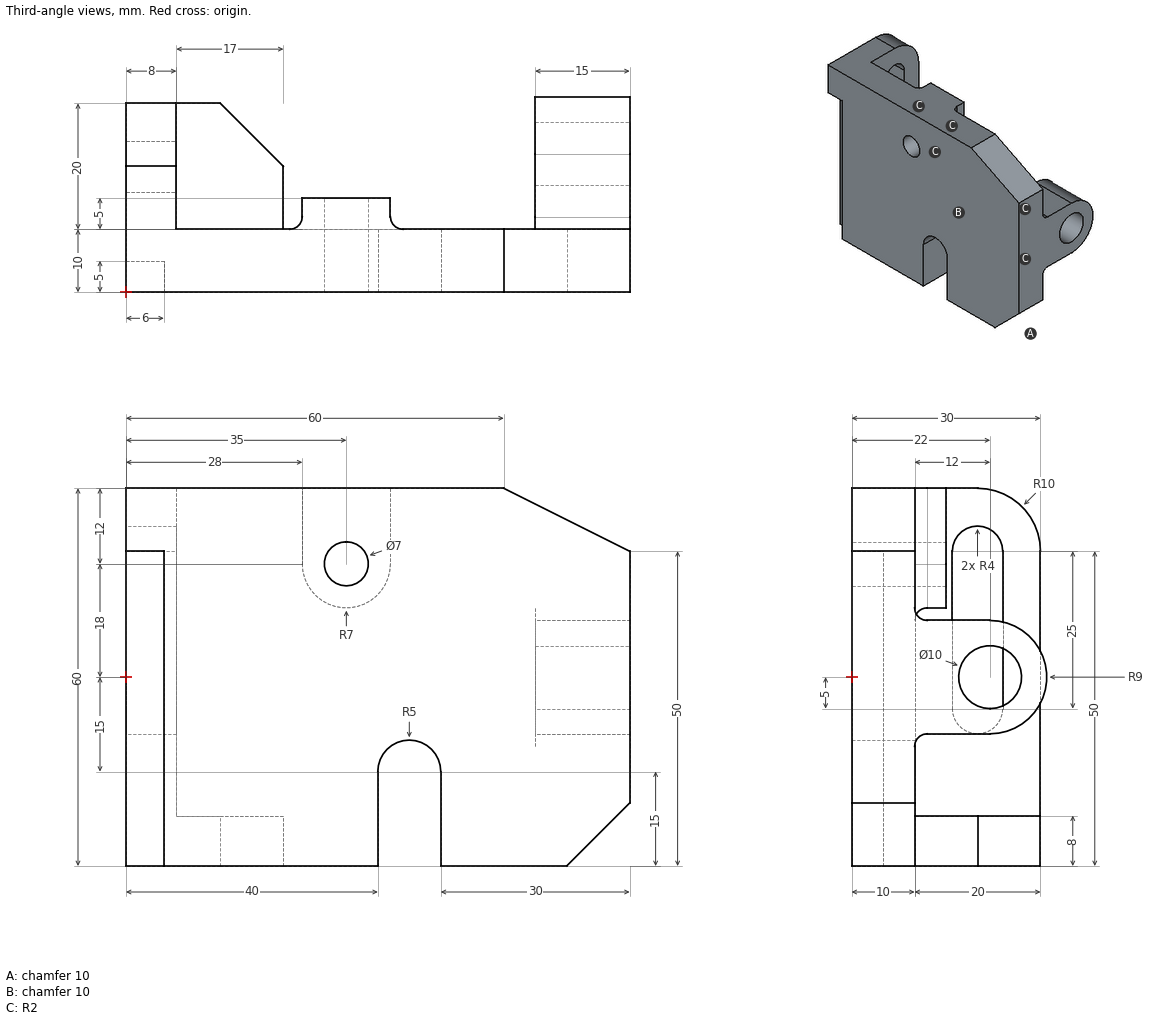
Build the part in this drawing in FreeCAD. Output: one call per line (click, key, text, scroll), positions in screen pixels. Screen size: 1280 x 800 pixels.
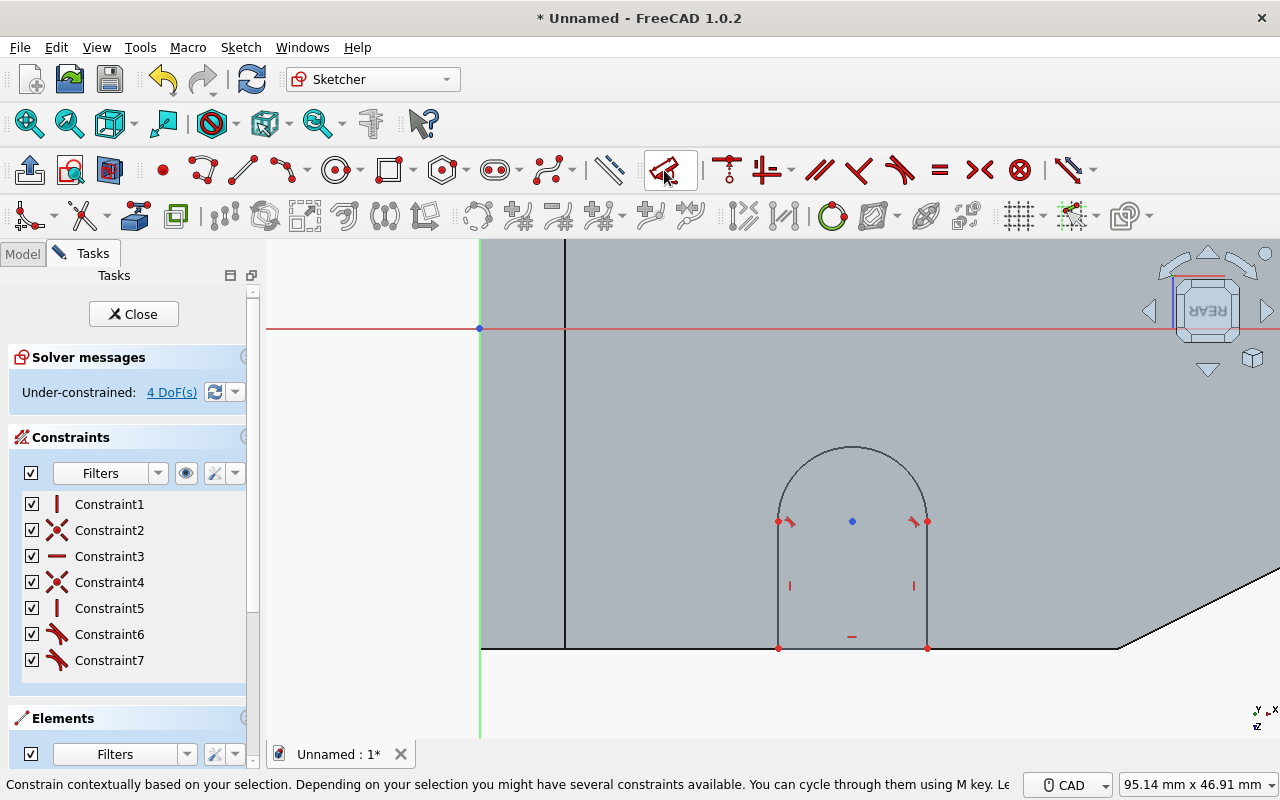
click(896, 461)
click(915, 435)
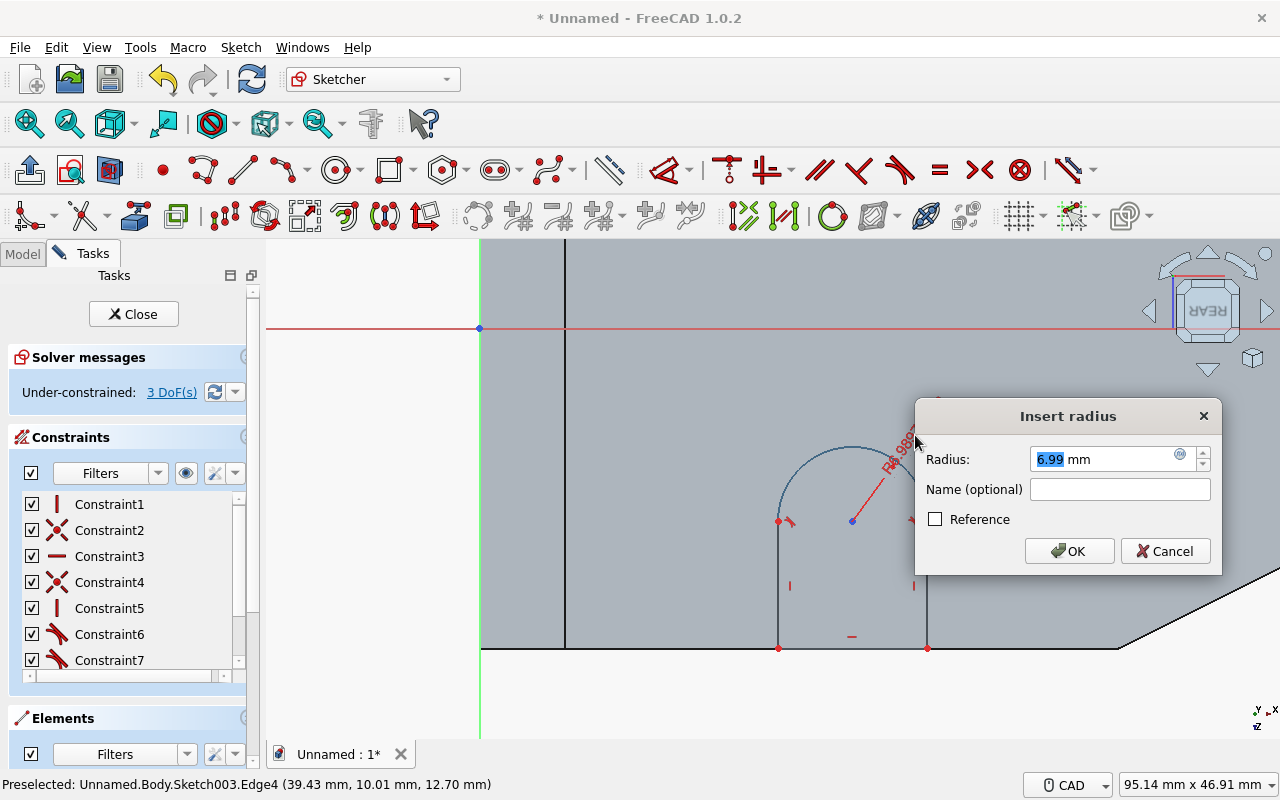
text(7)
key(Return)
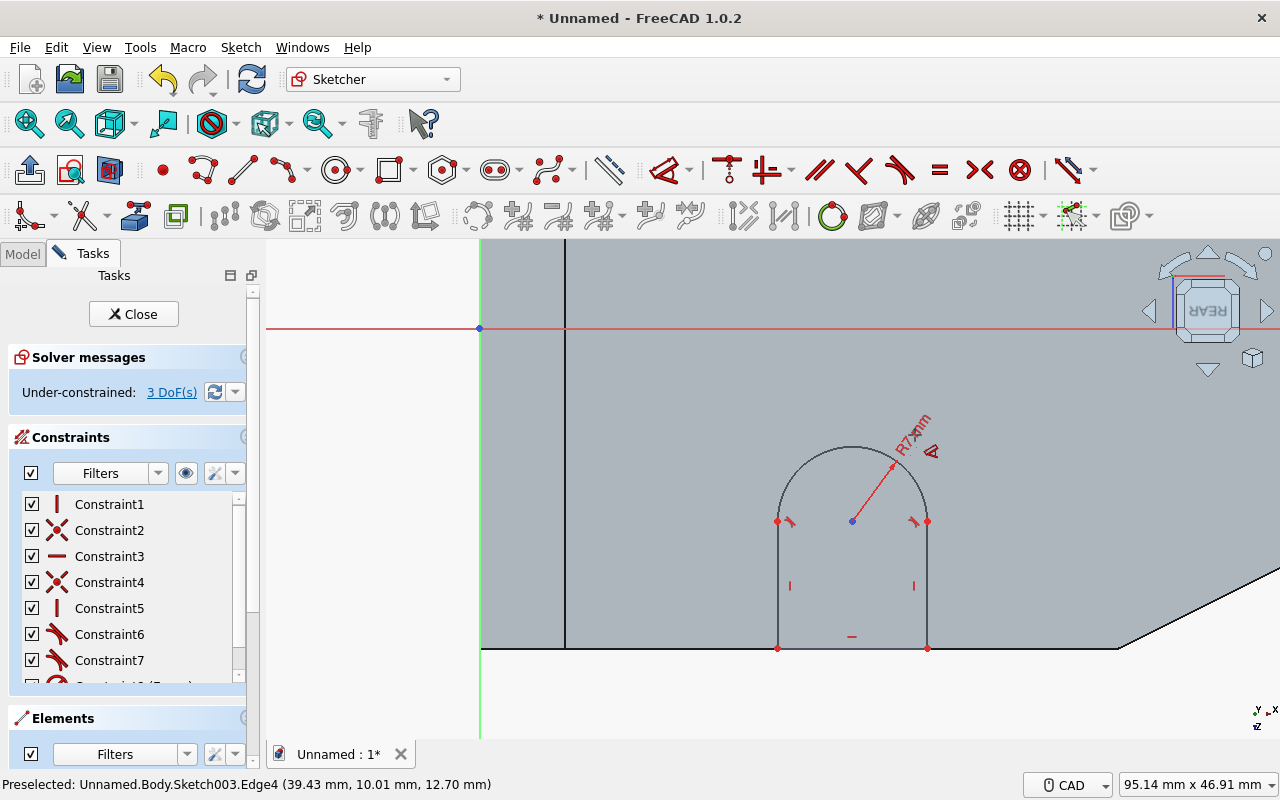
click(778, 560)
click(812, 585)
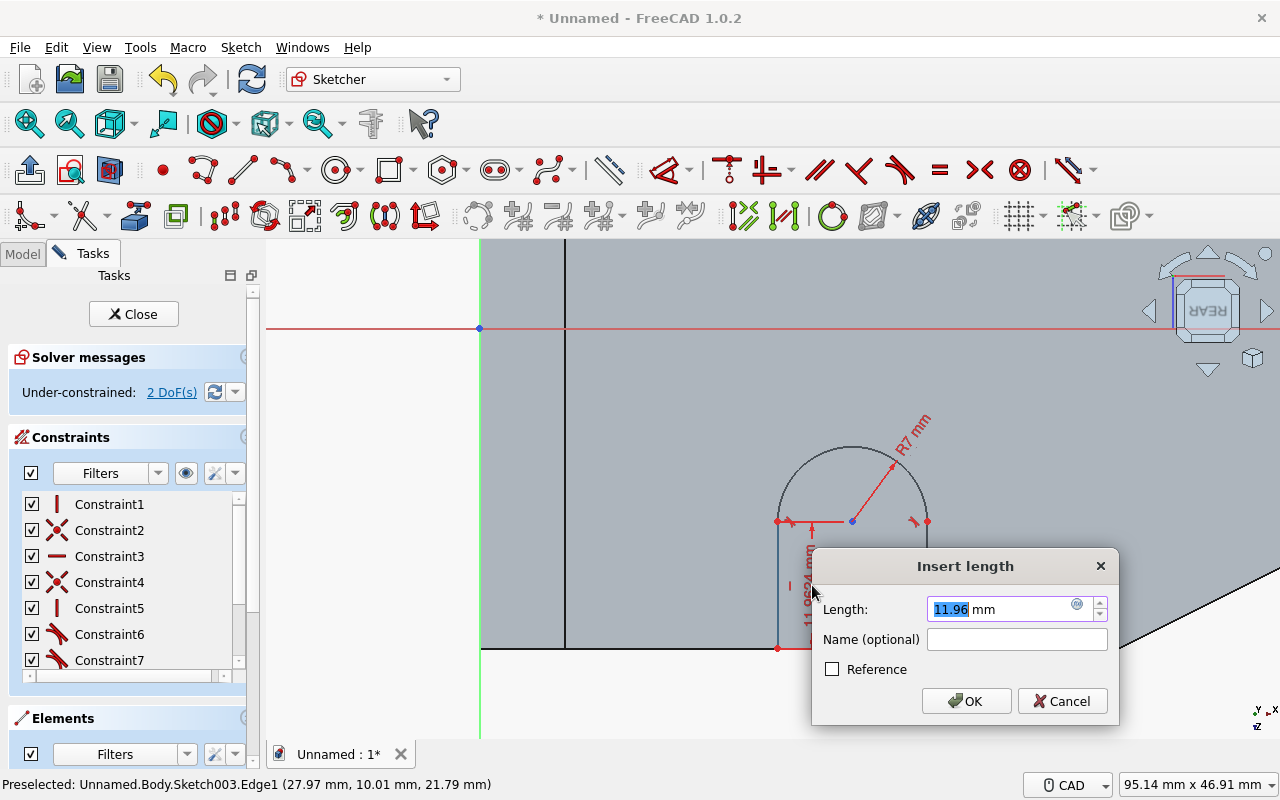
text(12)
key(Return)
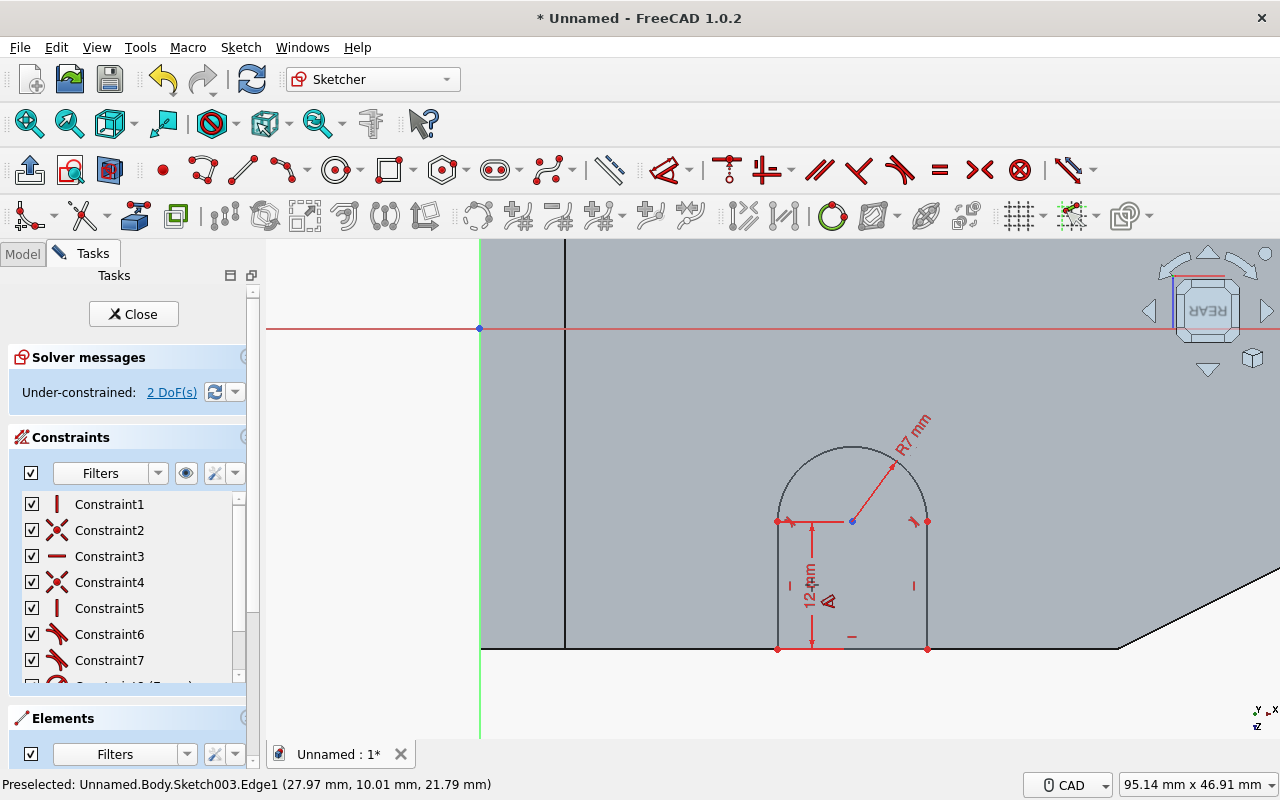
click(778, 522)
click(629, 295)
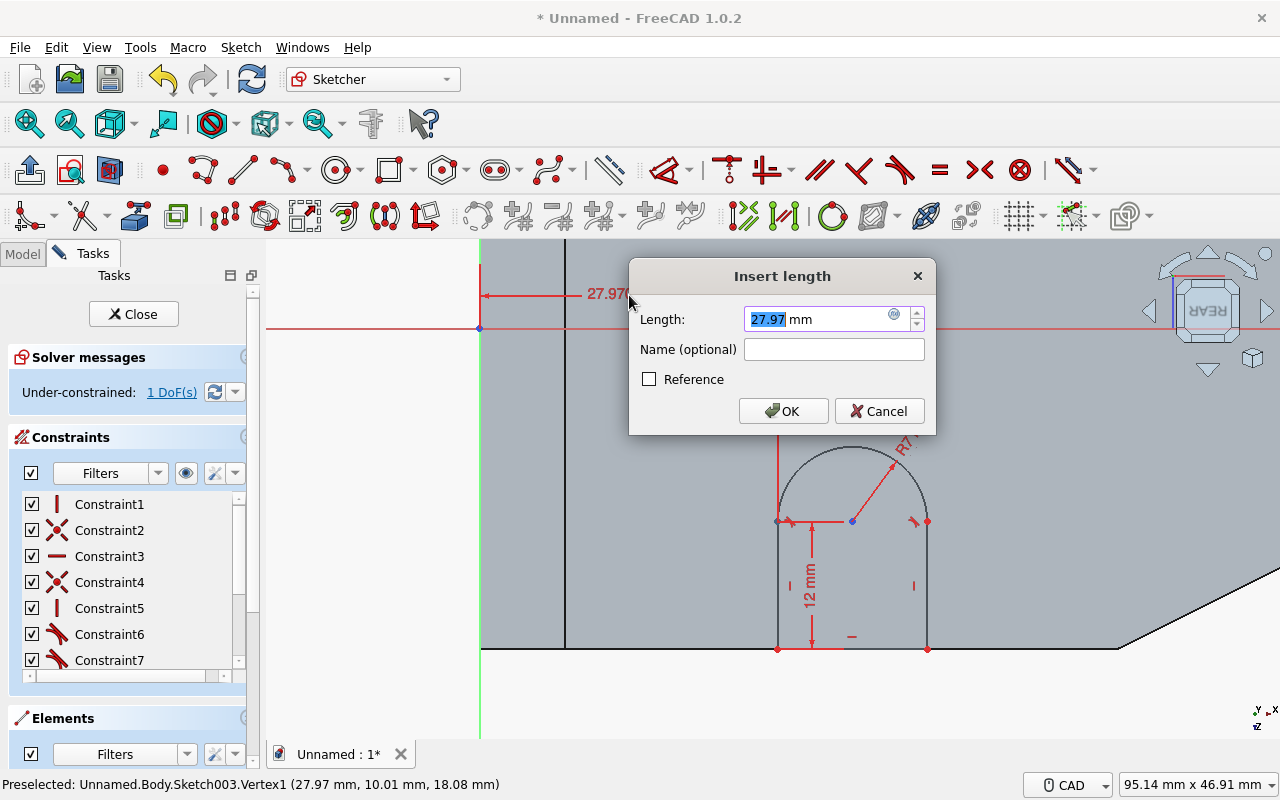
text(28)
key(Return)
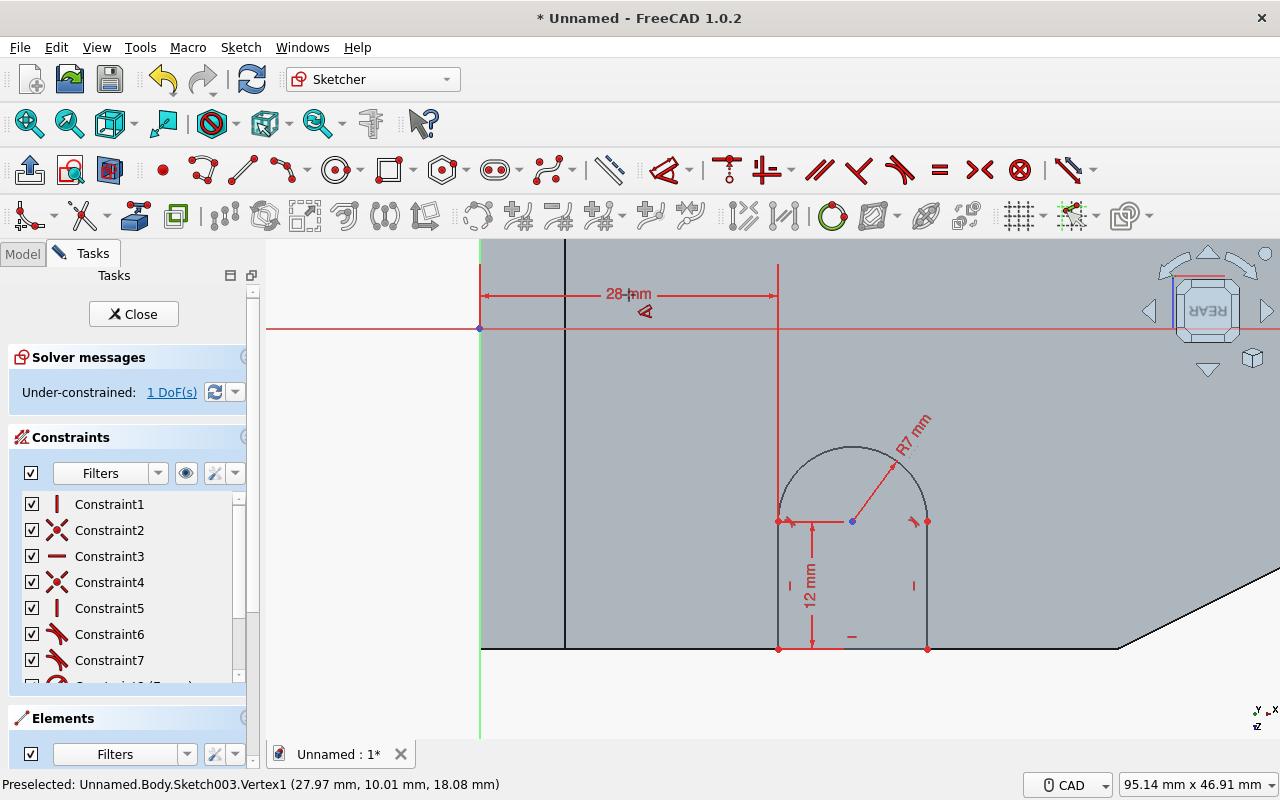
click(778, 522)
click(446, 425)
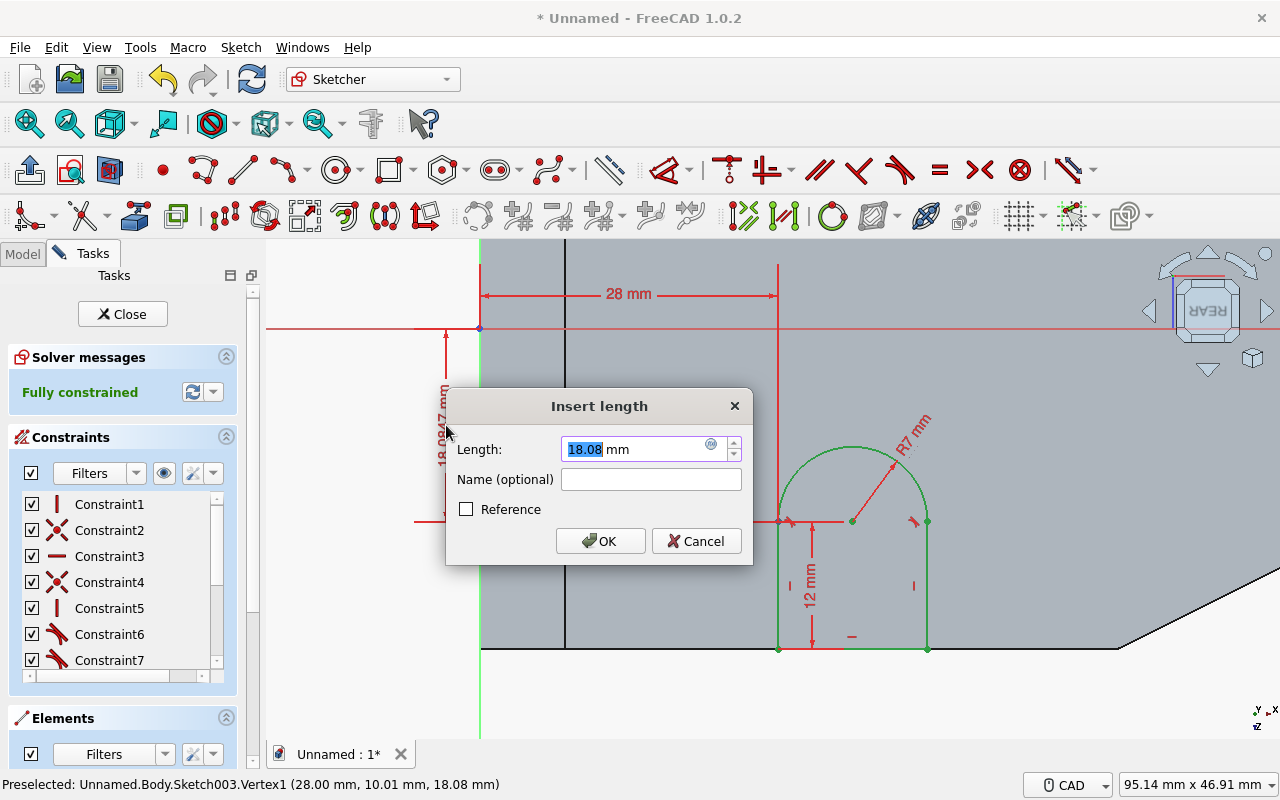
text(18)
key(Return)
key(Escape)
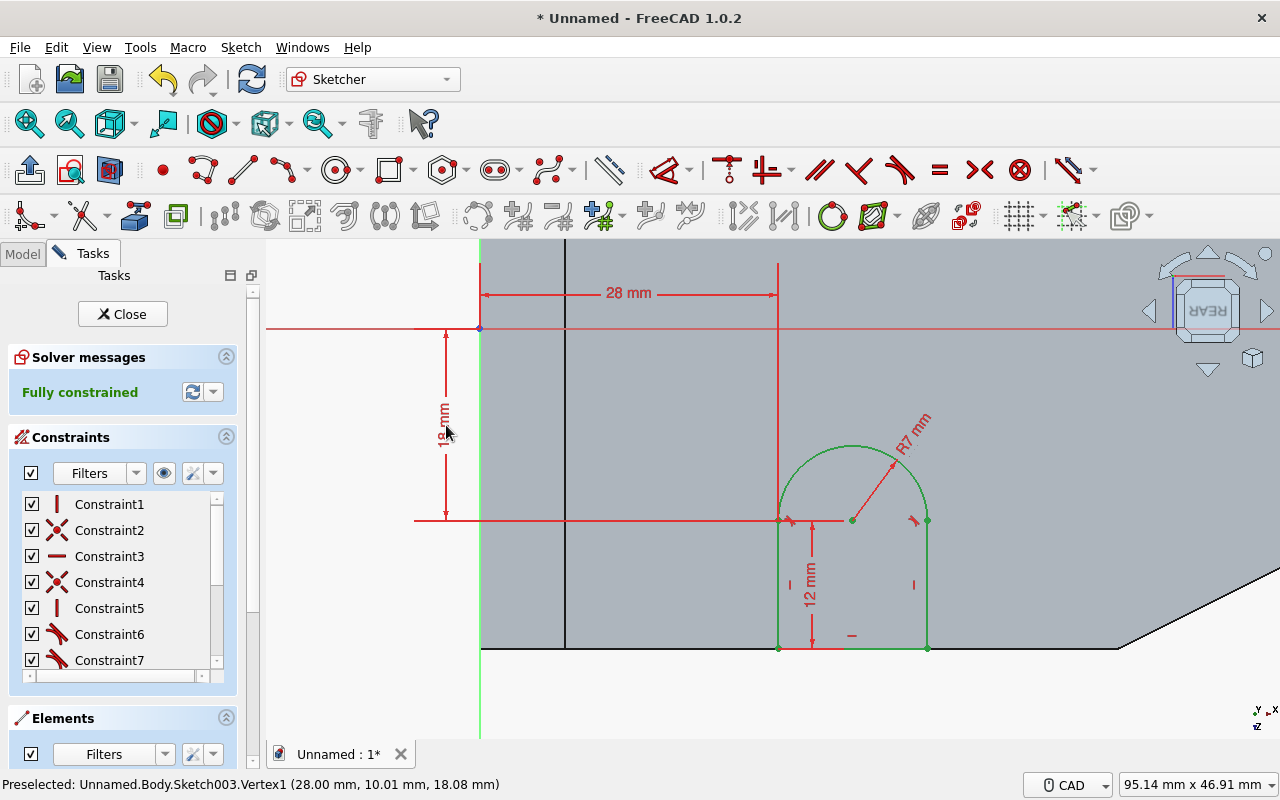
click(123, 314)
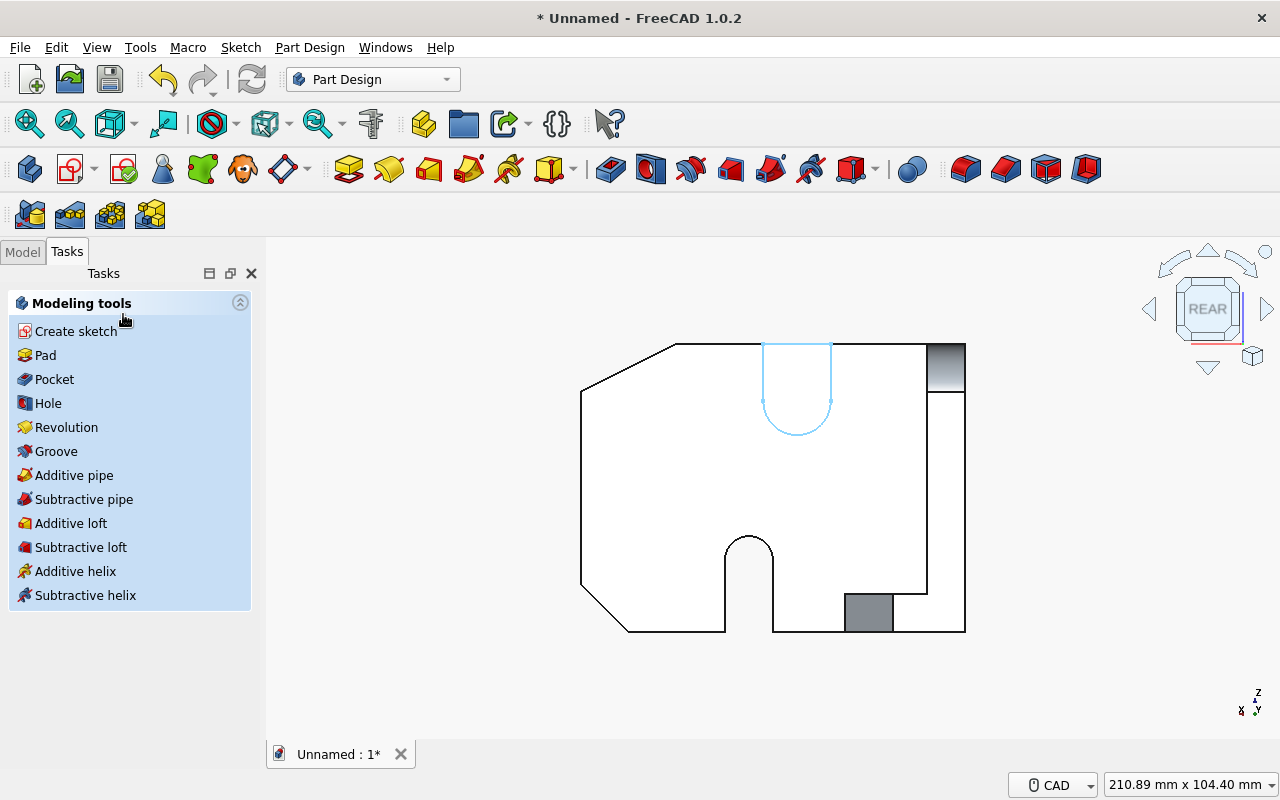
click(350, 170)